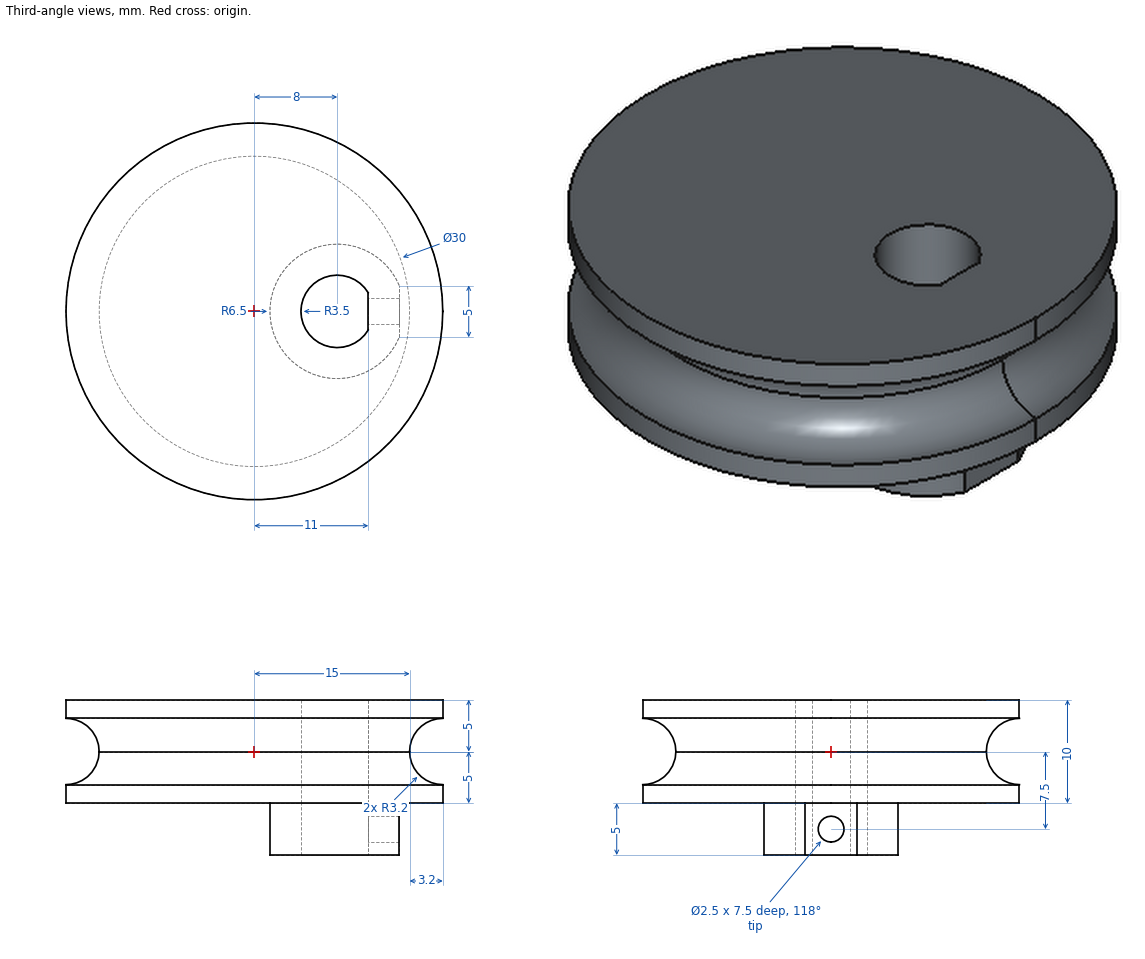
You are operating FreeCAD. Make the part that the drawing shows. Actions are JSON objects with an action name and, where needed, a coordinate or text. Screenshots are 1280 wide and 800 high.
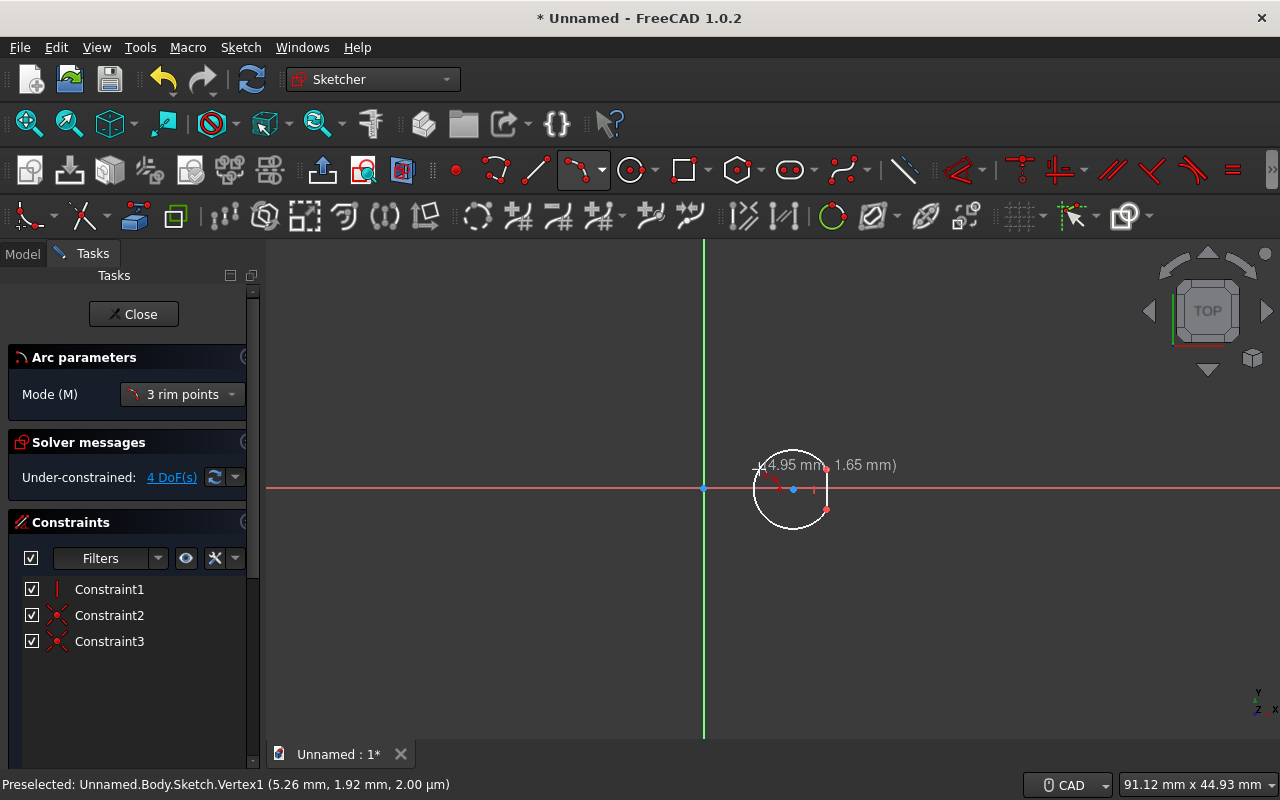
{"action": "left_click", "coordinate": [632, 170]}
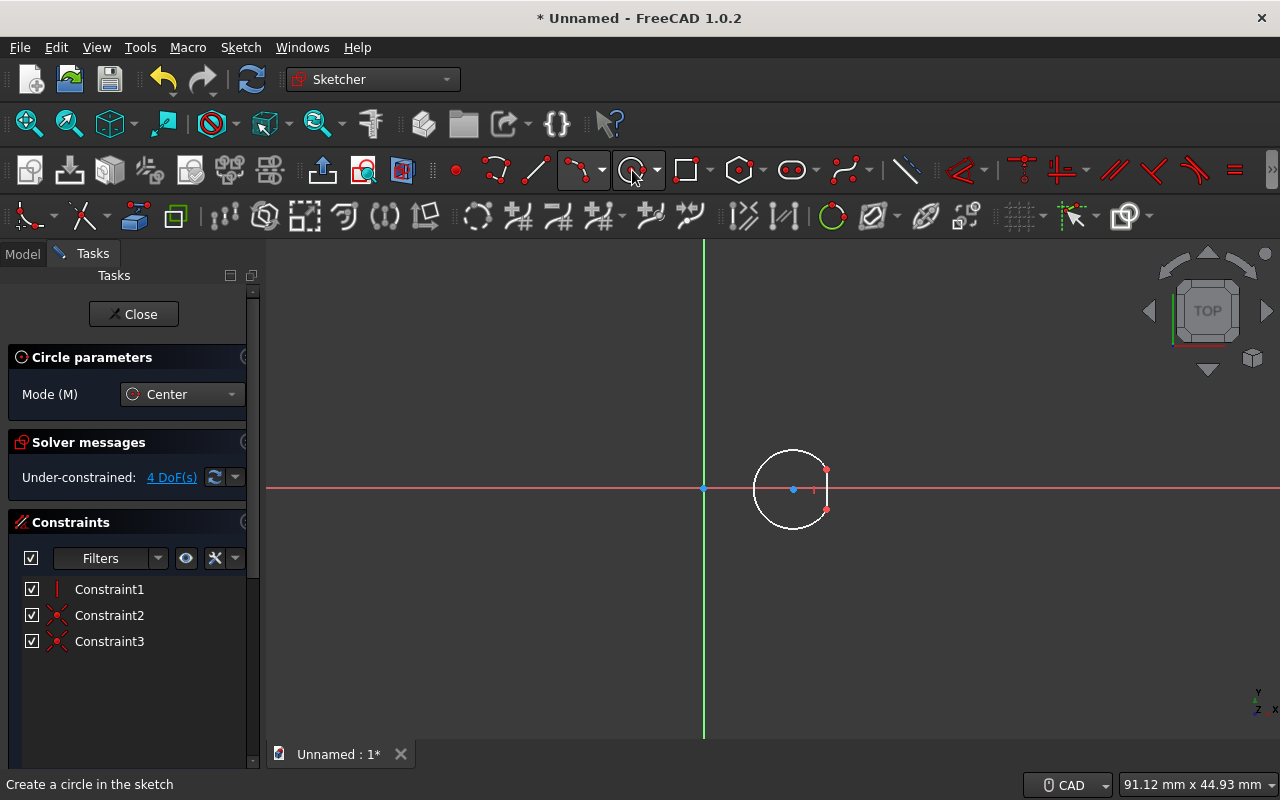
{"action": "left_click", "coordinate": [704, 488]}
{"action": "mouse_move", "coordinate": [822, 370]}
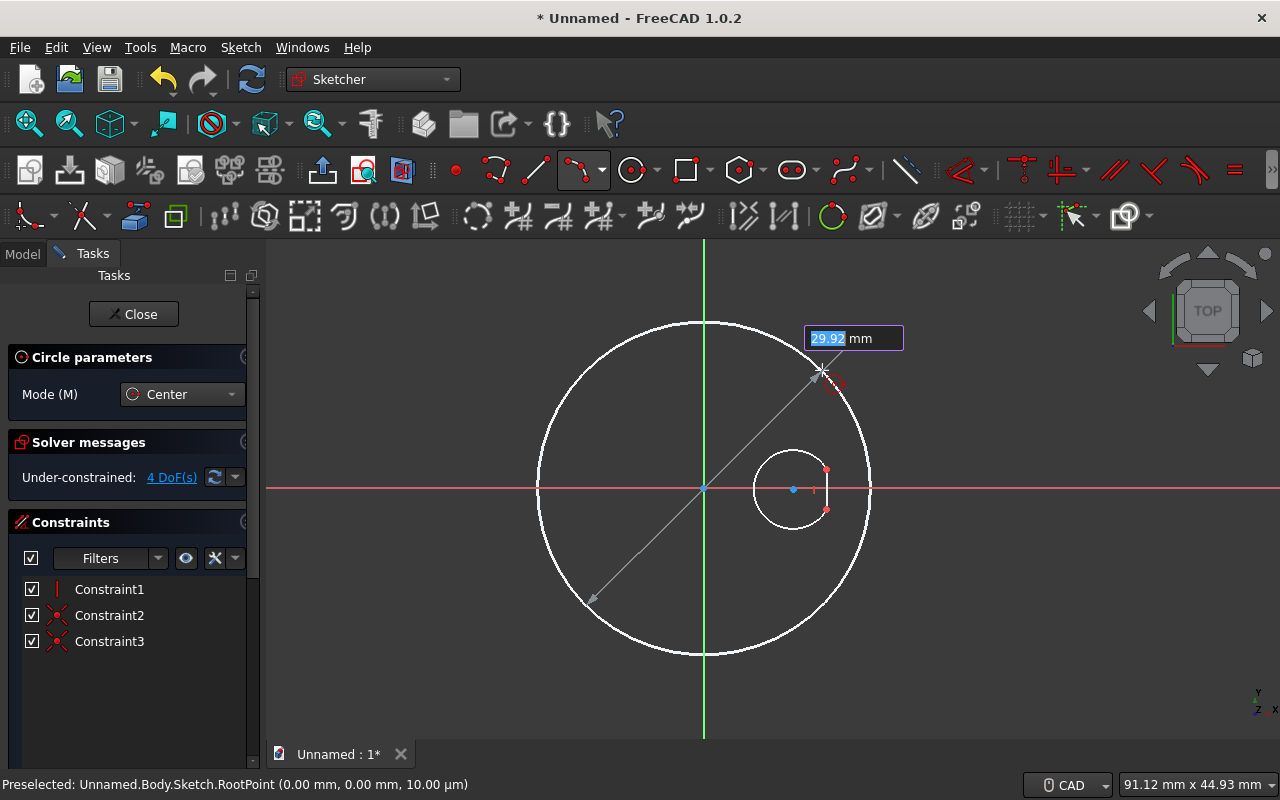
{"action": "type", "text": "30"}
{"action": "key", "text": "Return"}
{"action": "key", "text": "Escape"}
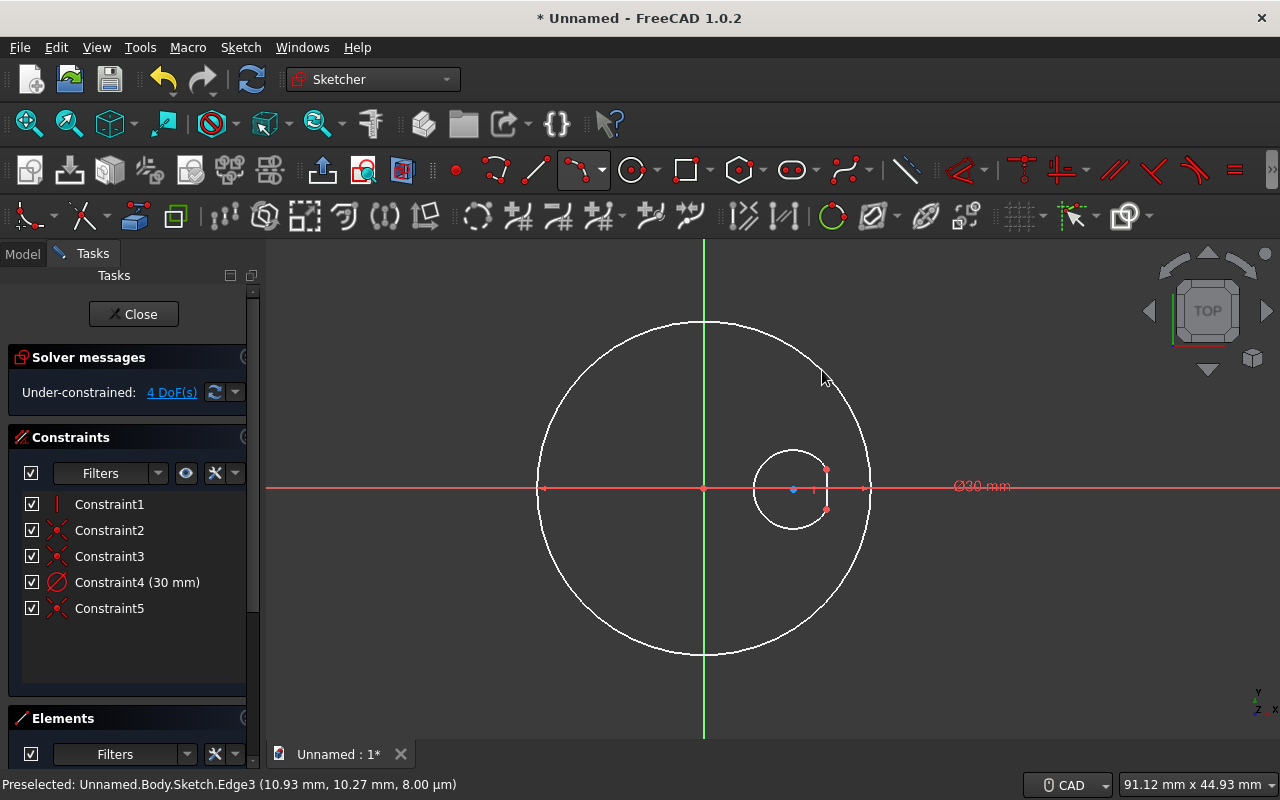
{"action": "left_click", "coordinate": [793, 489]}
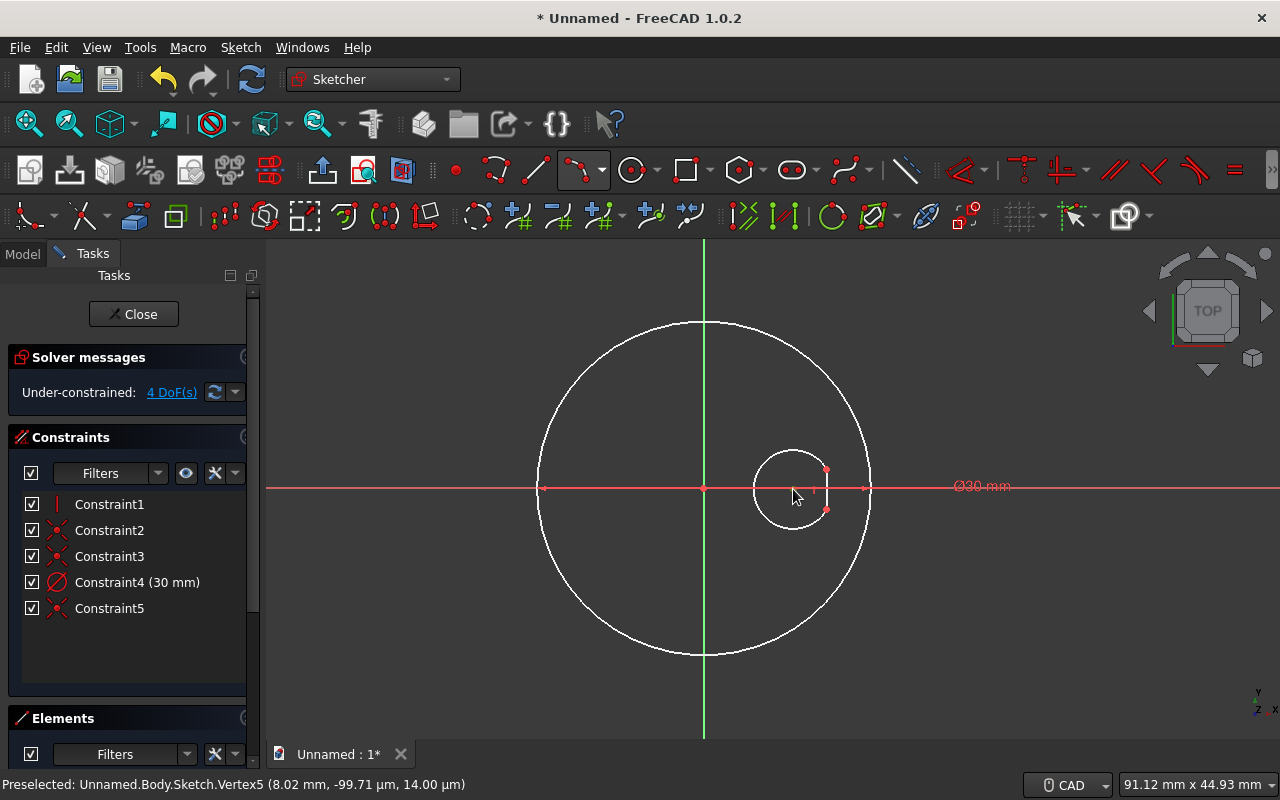
{"action": "left_click", "coordinate": [353, 488]}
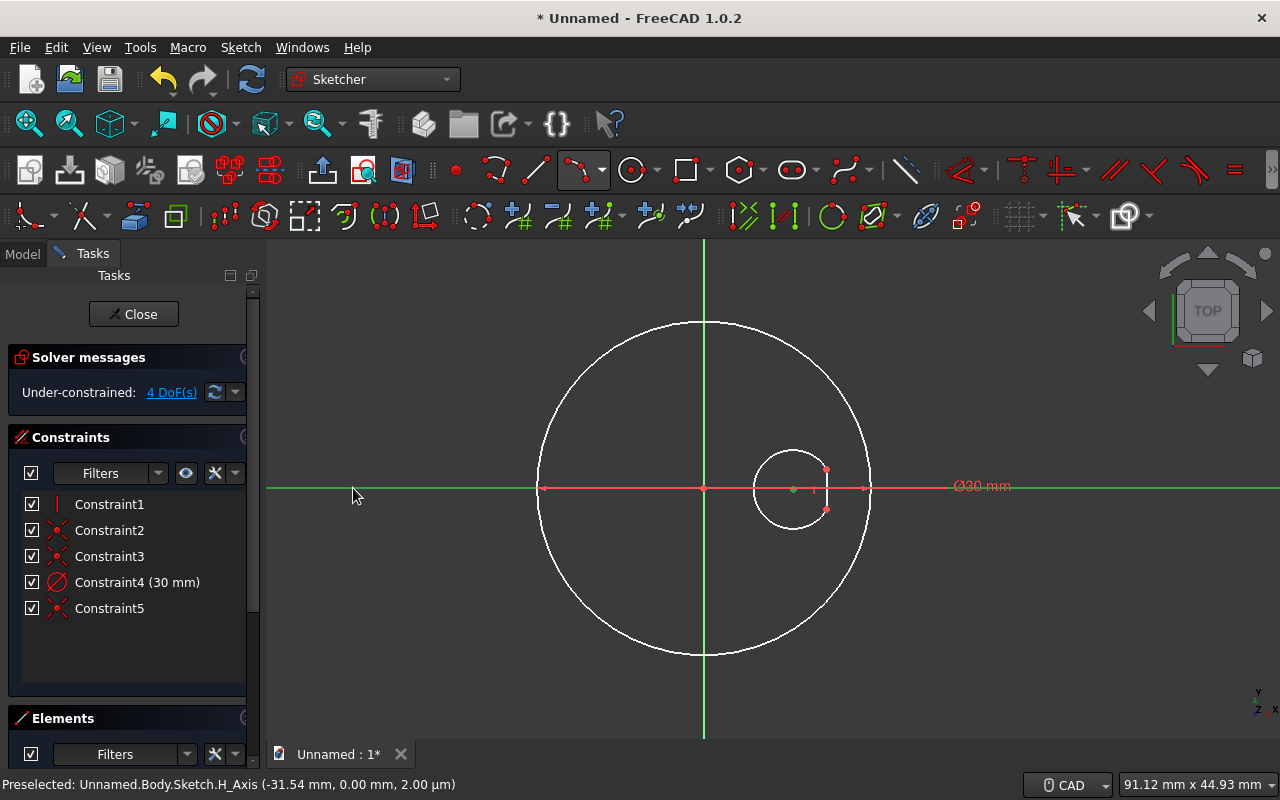
{"action": "left_click", "coordinate": [1022, 170]}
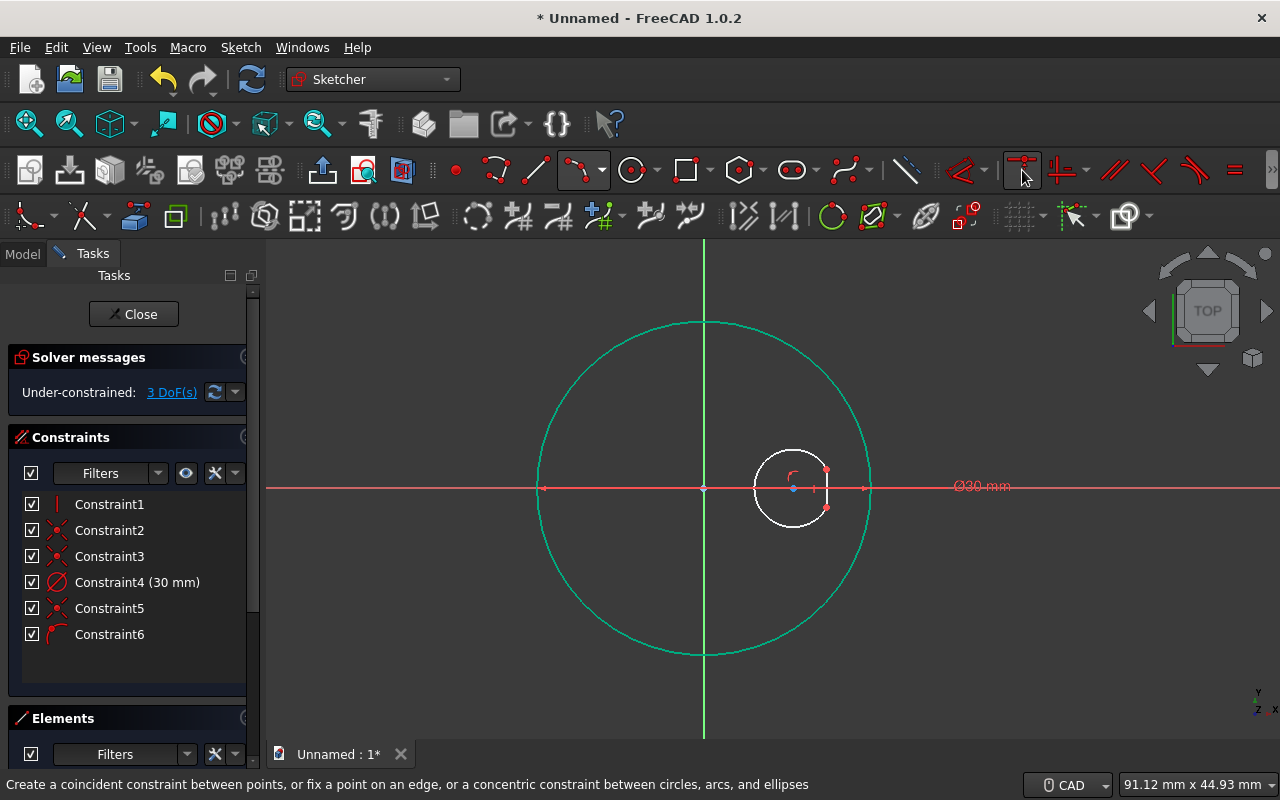
{"action": "left_click", "coordinate": [960, 170]}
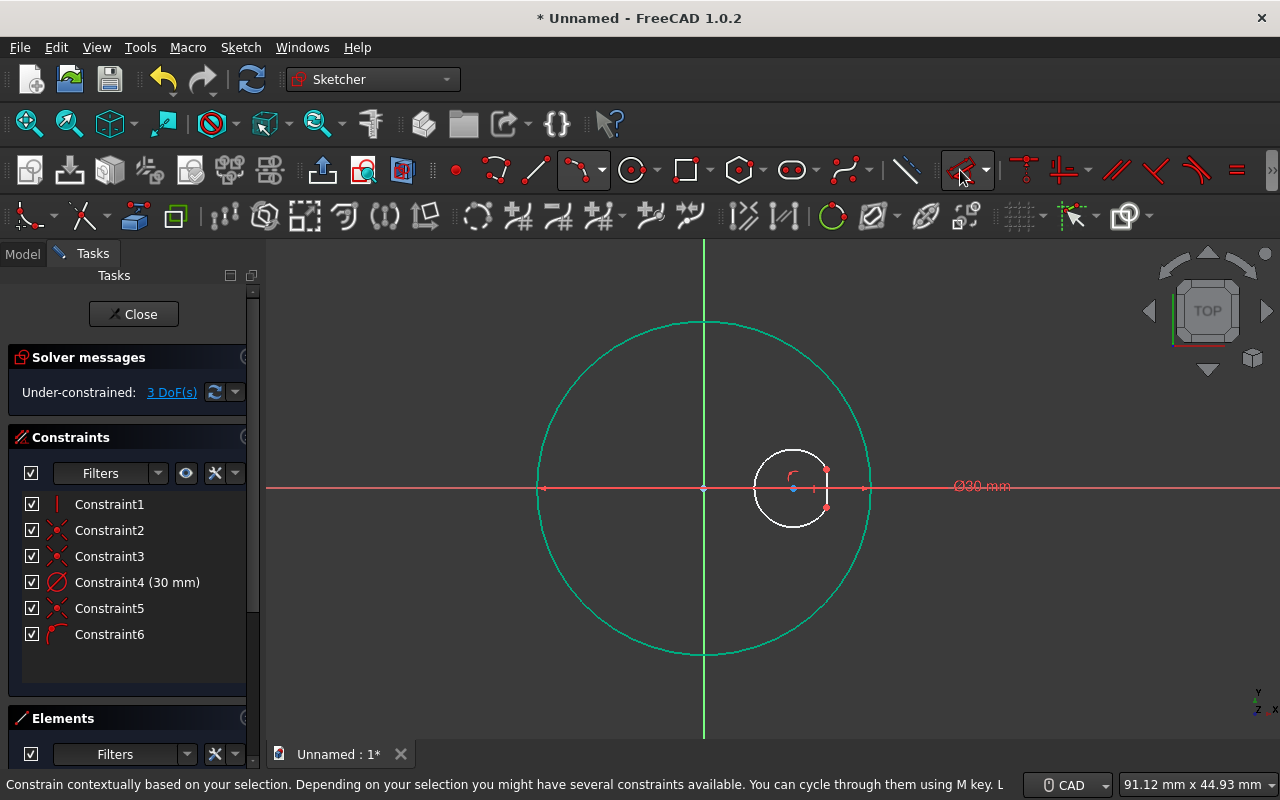
{"action": "left_click", "coordinate": [774, 455]}
{"action": "left_click", "coordinate": [758, 427]}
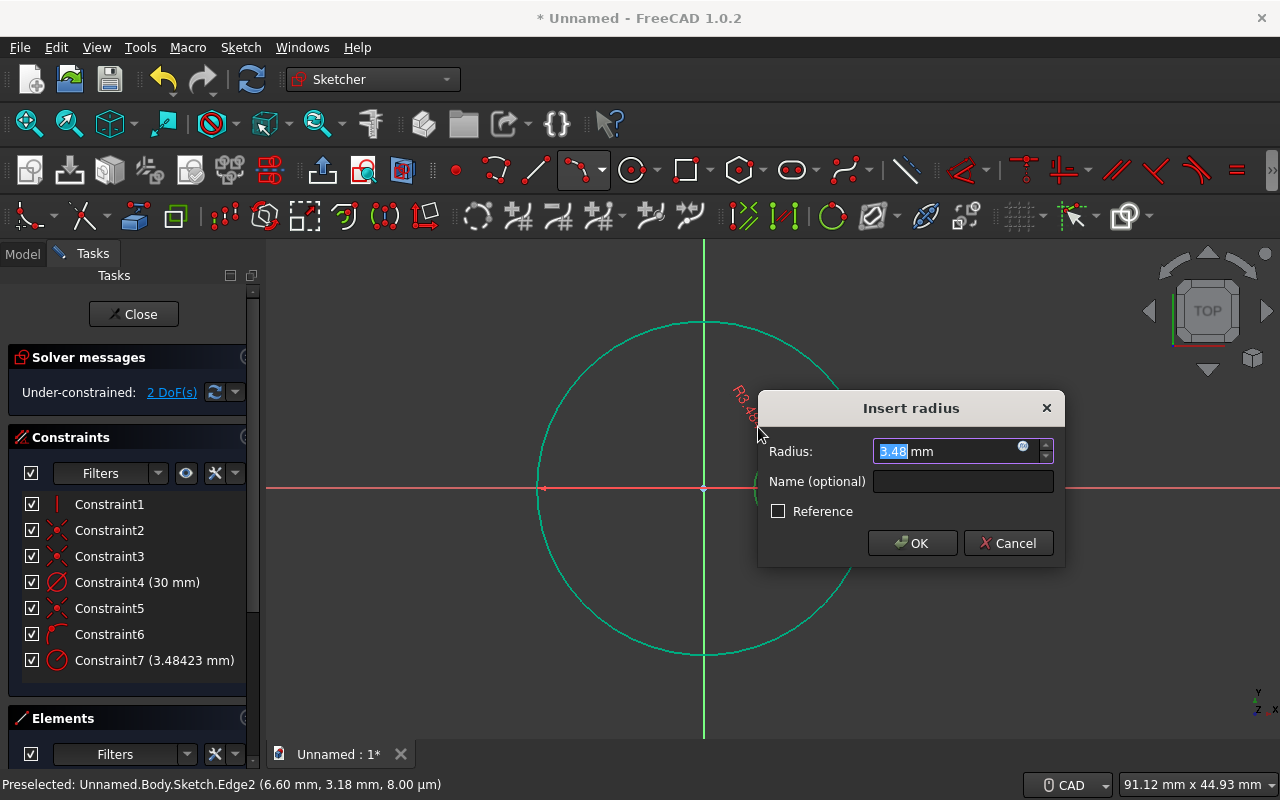
{"action": "type", "text": "3.5"}
{"action": "key", "text": "Return"}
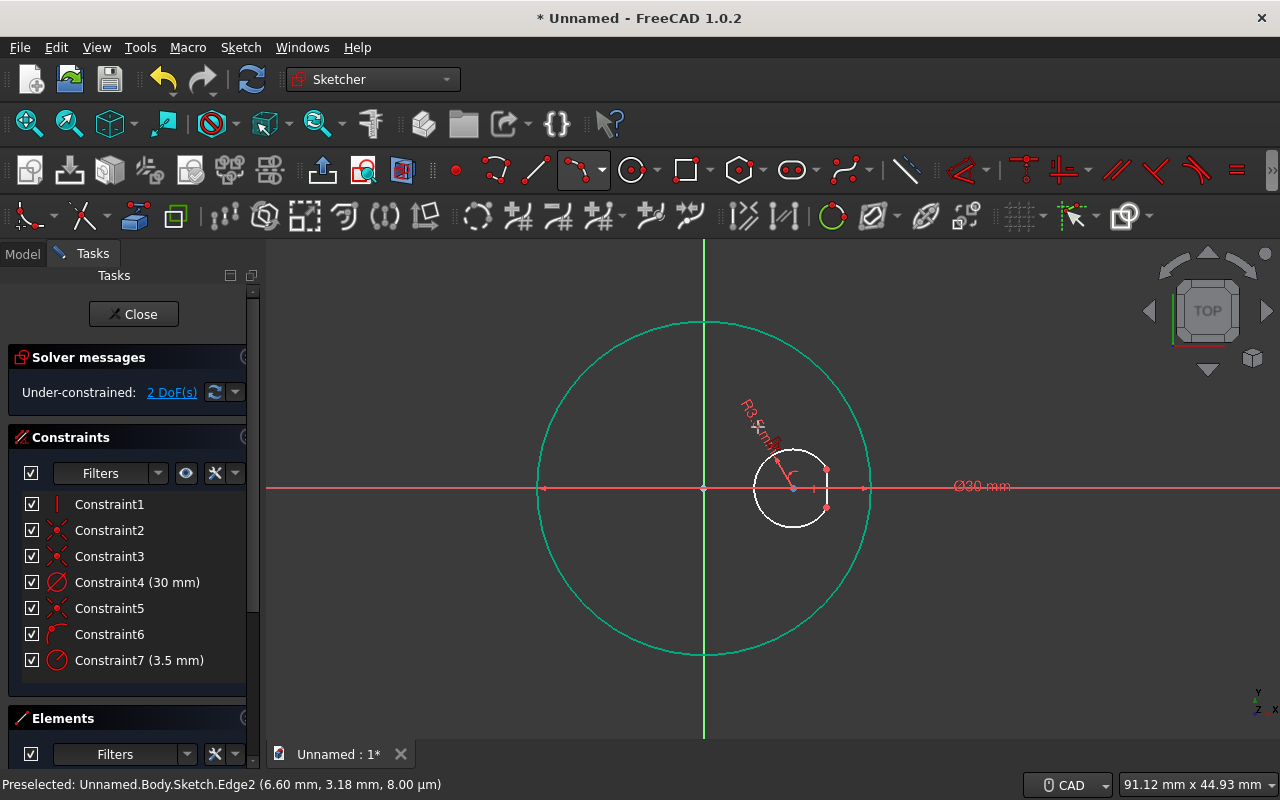
{"action": "left_click", "coordinate": [793, 488]}
{"action": "left_click", "coordinate": [749, 522]}